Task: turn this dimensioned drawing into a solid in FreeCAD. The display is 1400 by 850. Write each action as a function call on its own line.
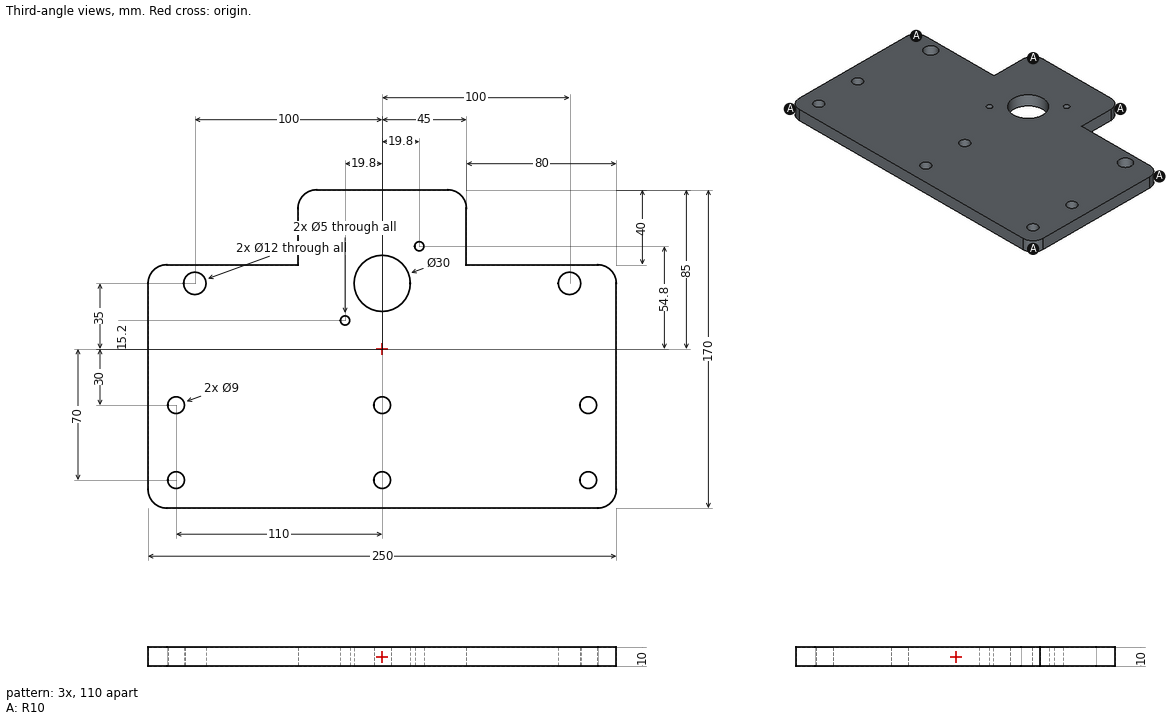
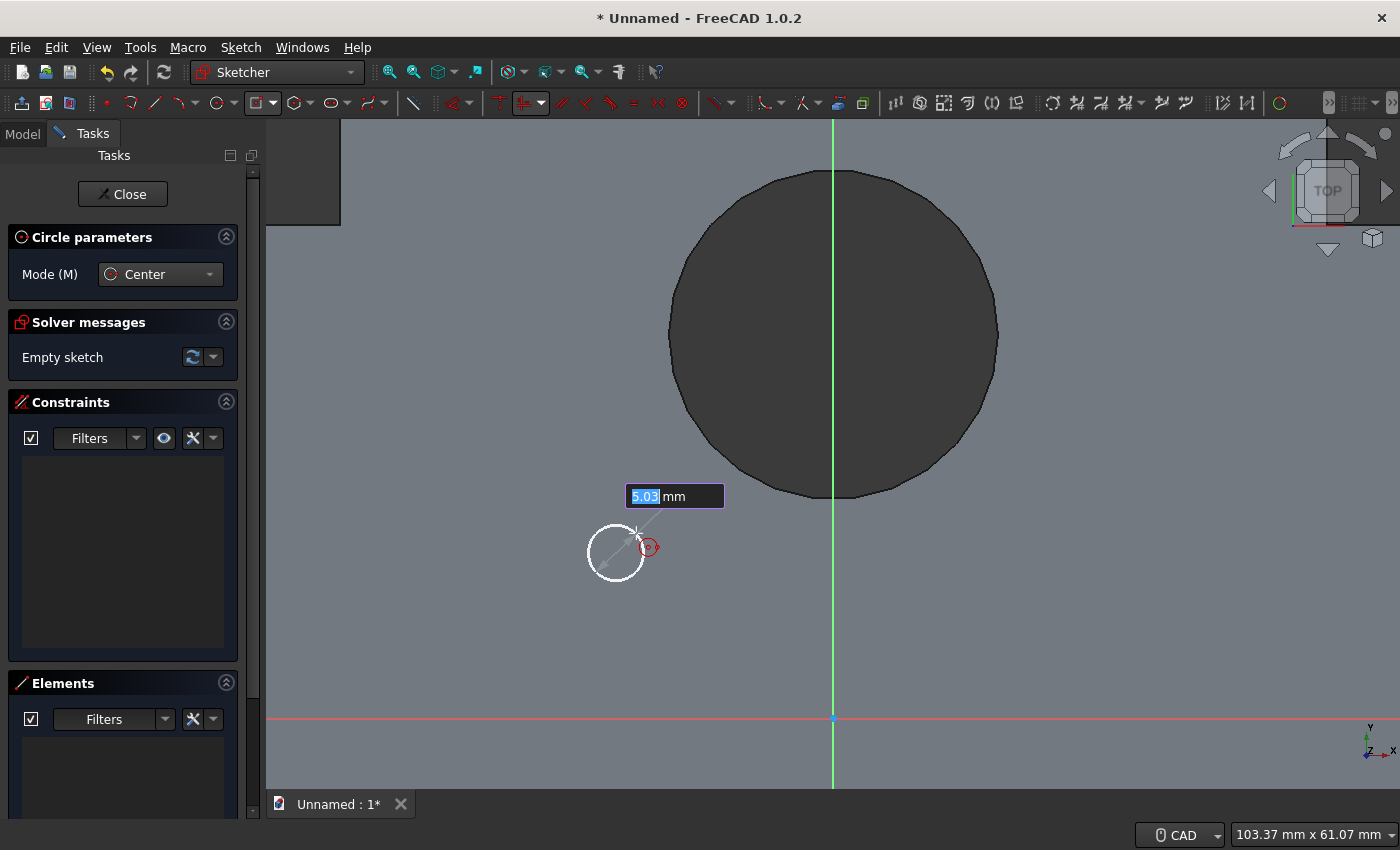
text(5)
key(Return)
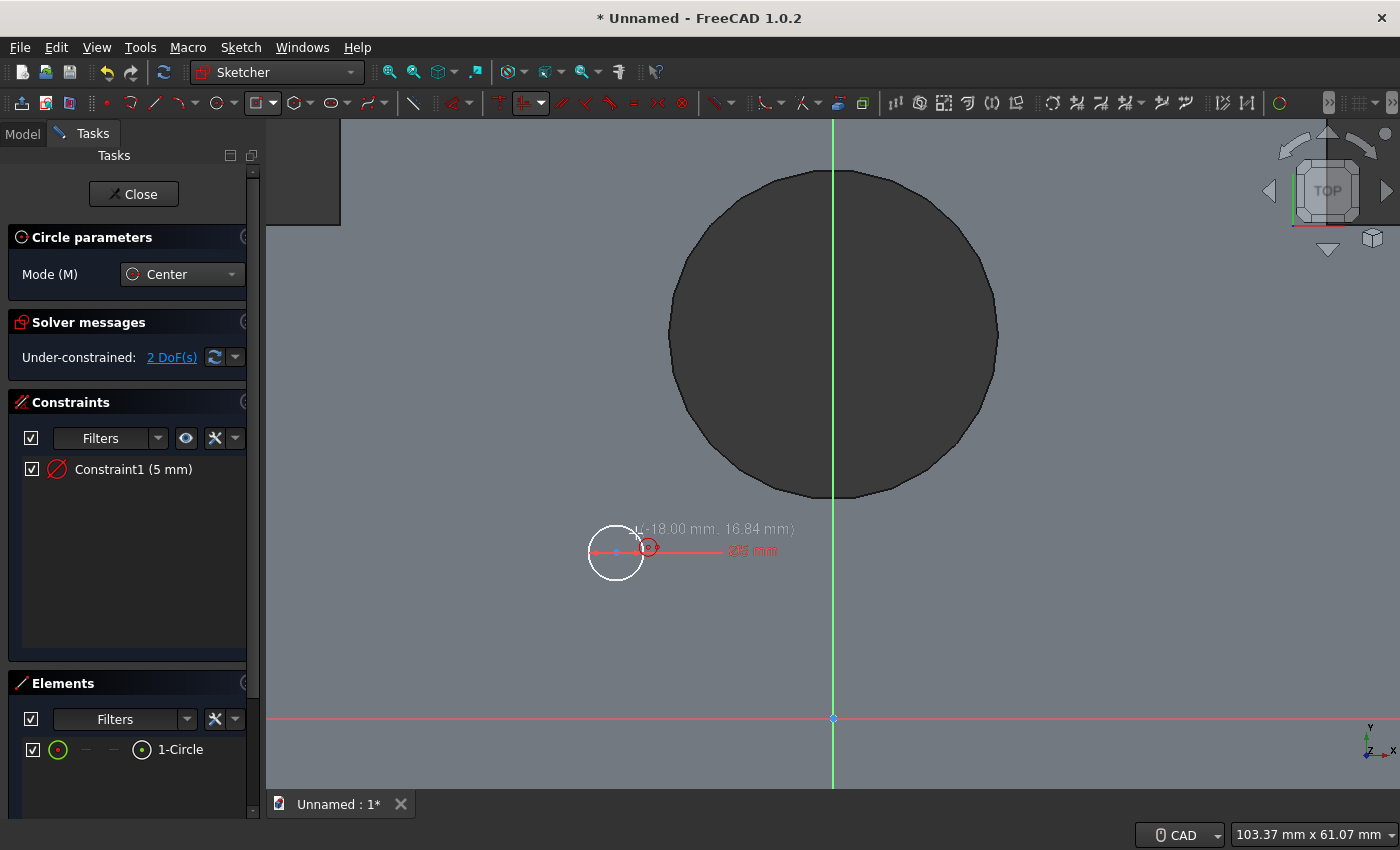
scroll(624, 555, down, 2)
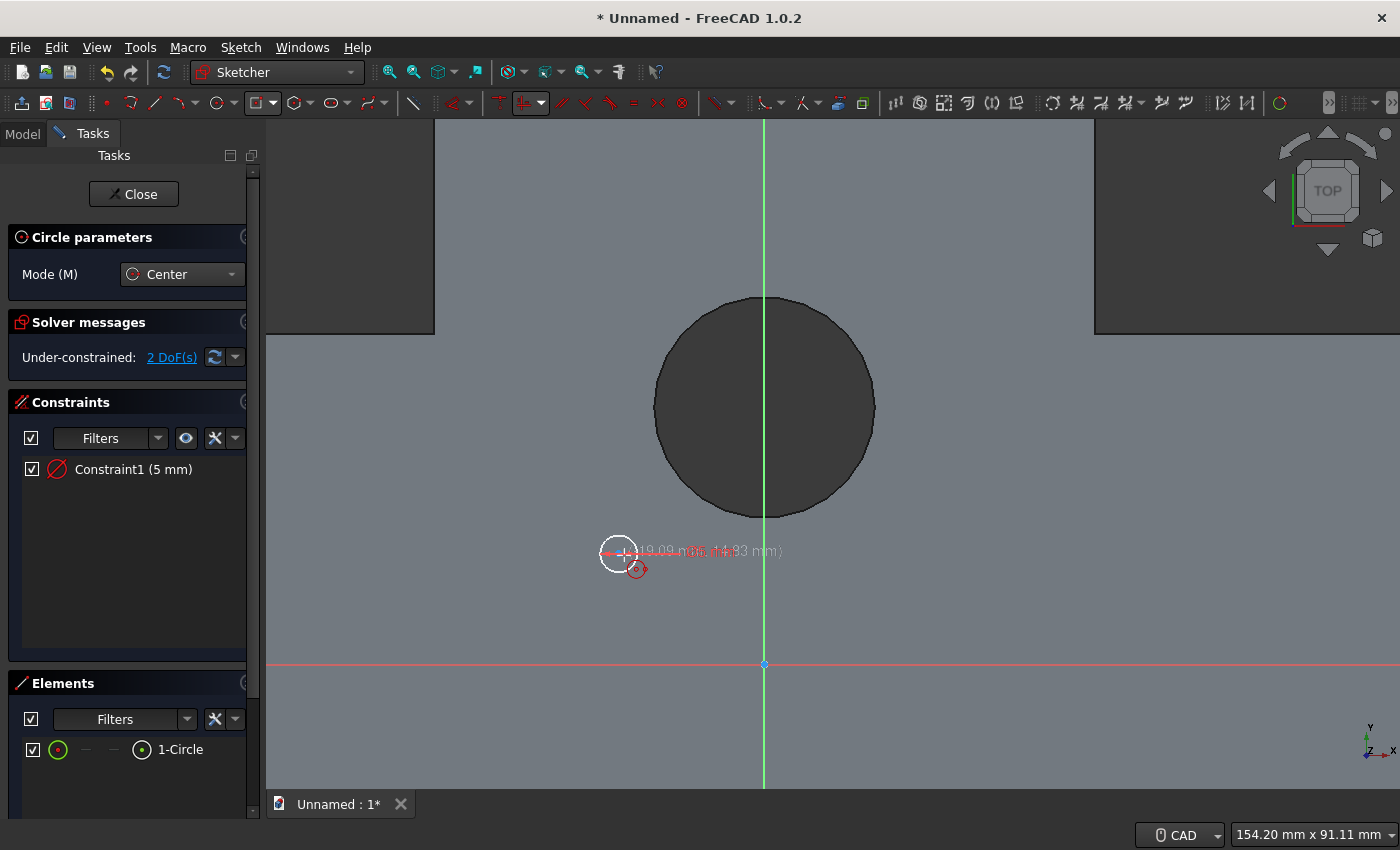
scroll(910, 262, up, 2)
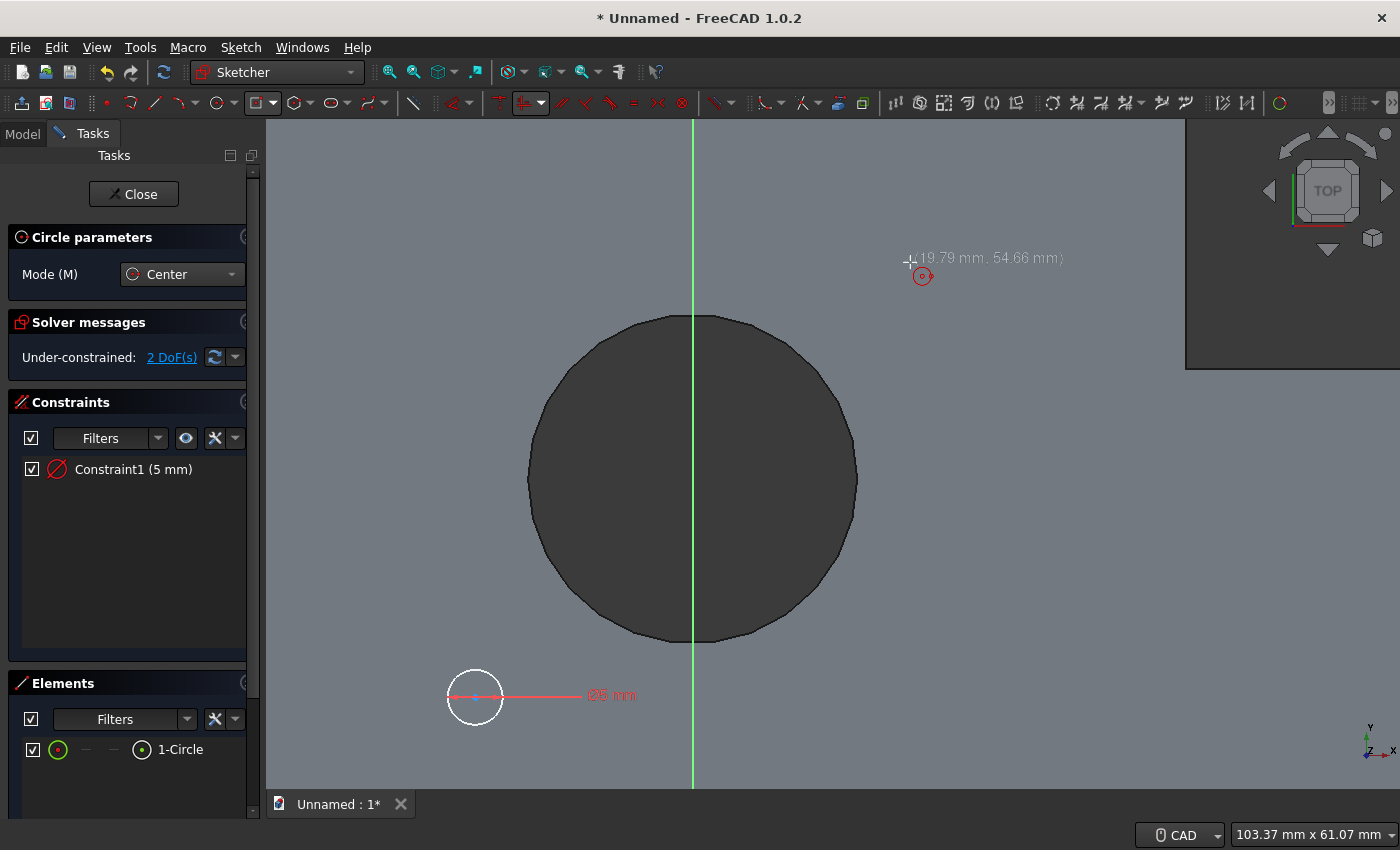
click(910, 262)
move(929, 242)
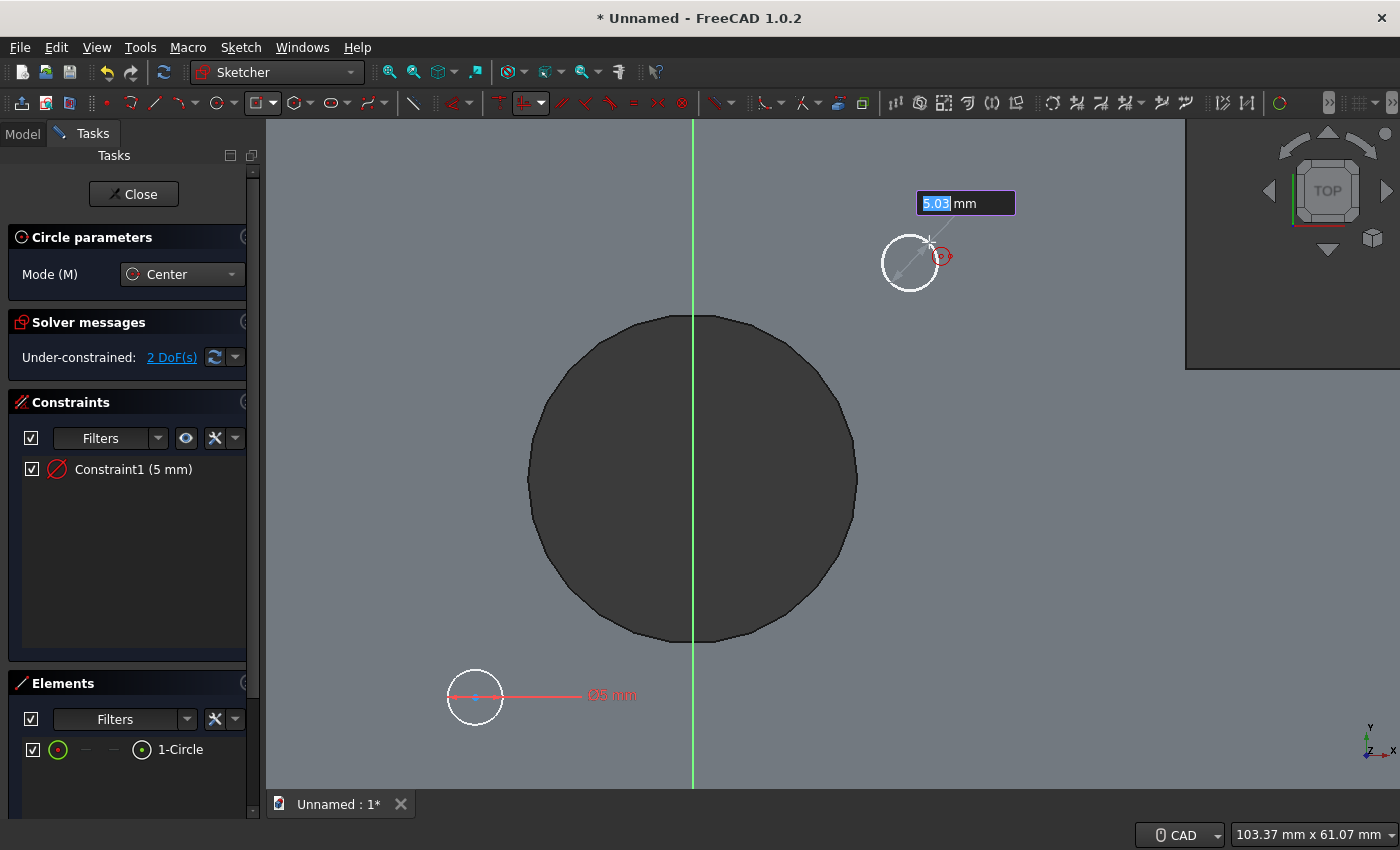
text(5)
key(Return)
key(Escape)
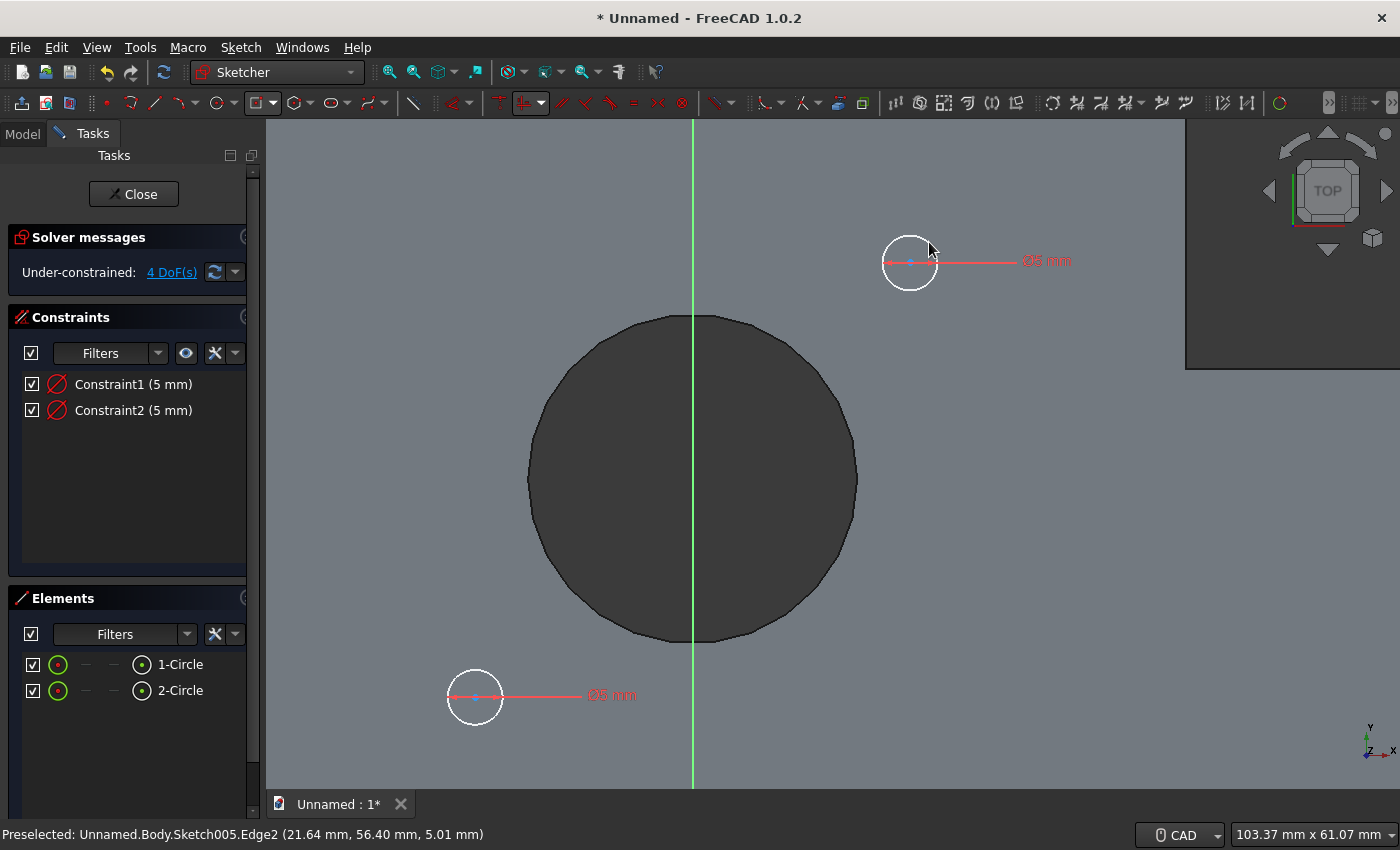
click(452, 104)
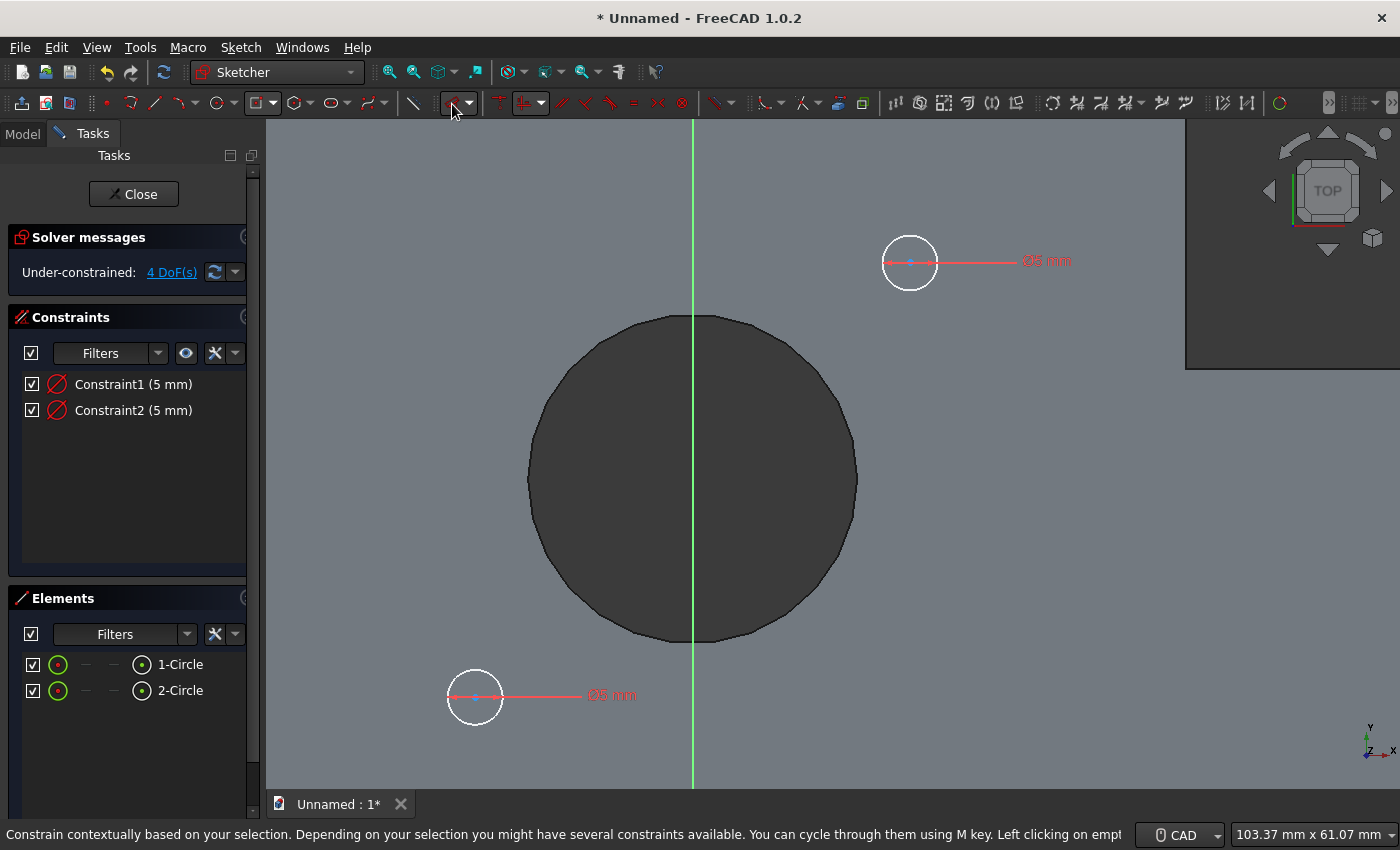
click(475, 697)
click(584, 663)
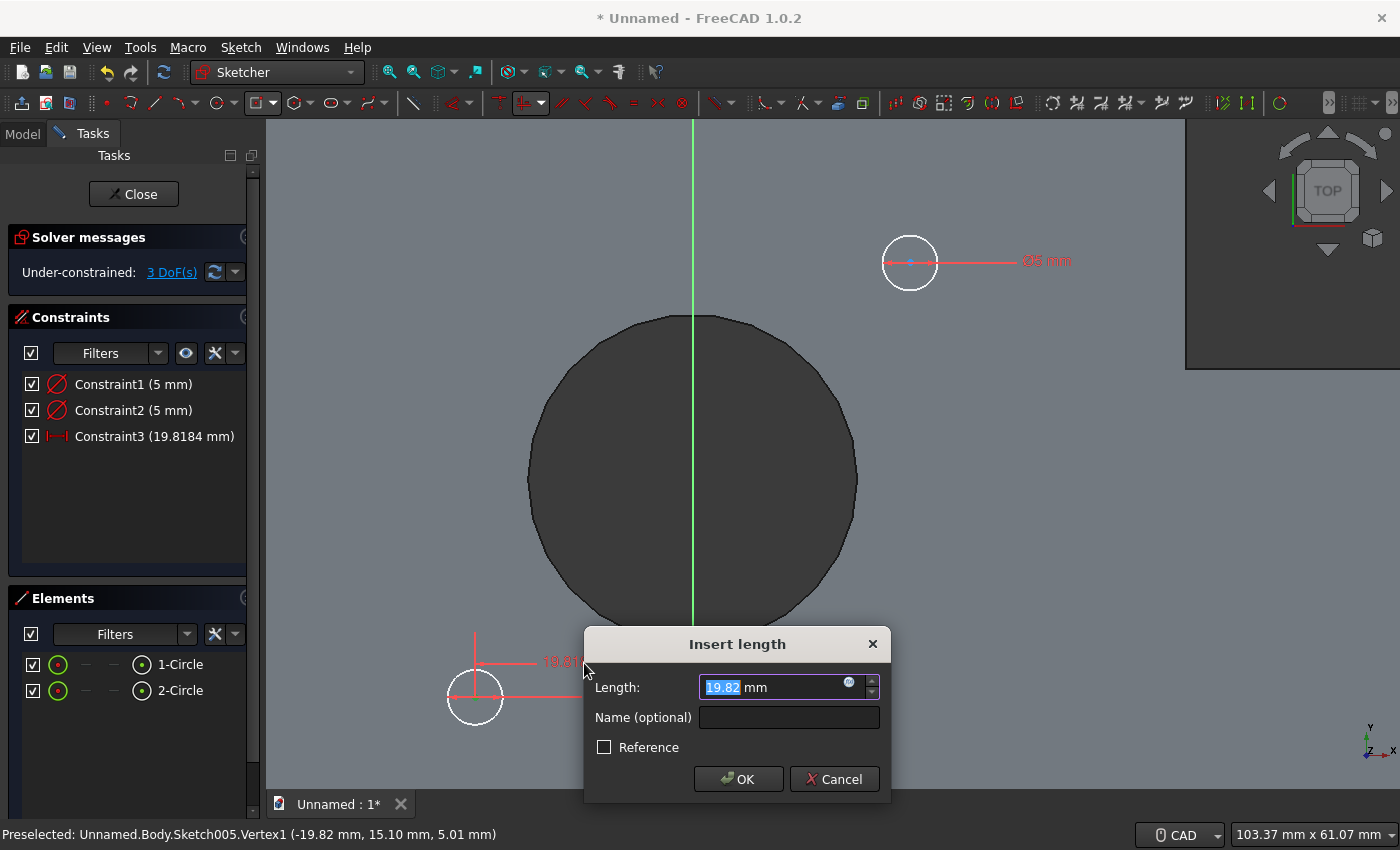
text(19.8)
key(Return)